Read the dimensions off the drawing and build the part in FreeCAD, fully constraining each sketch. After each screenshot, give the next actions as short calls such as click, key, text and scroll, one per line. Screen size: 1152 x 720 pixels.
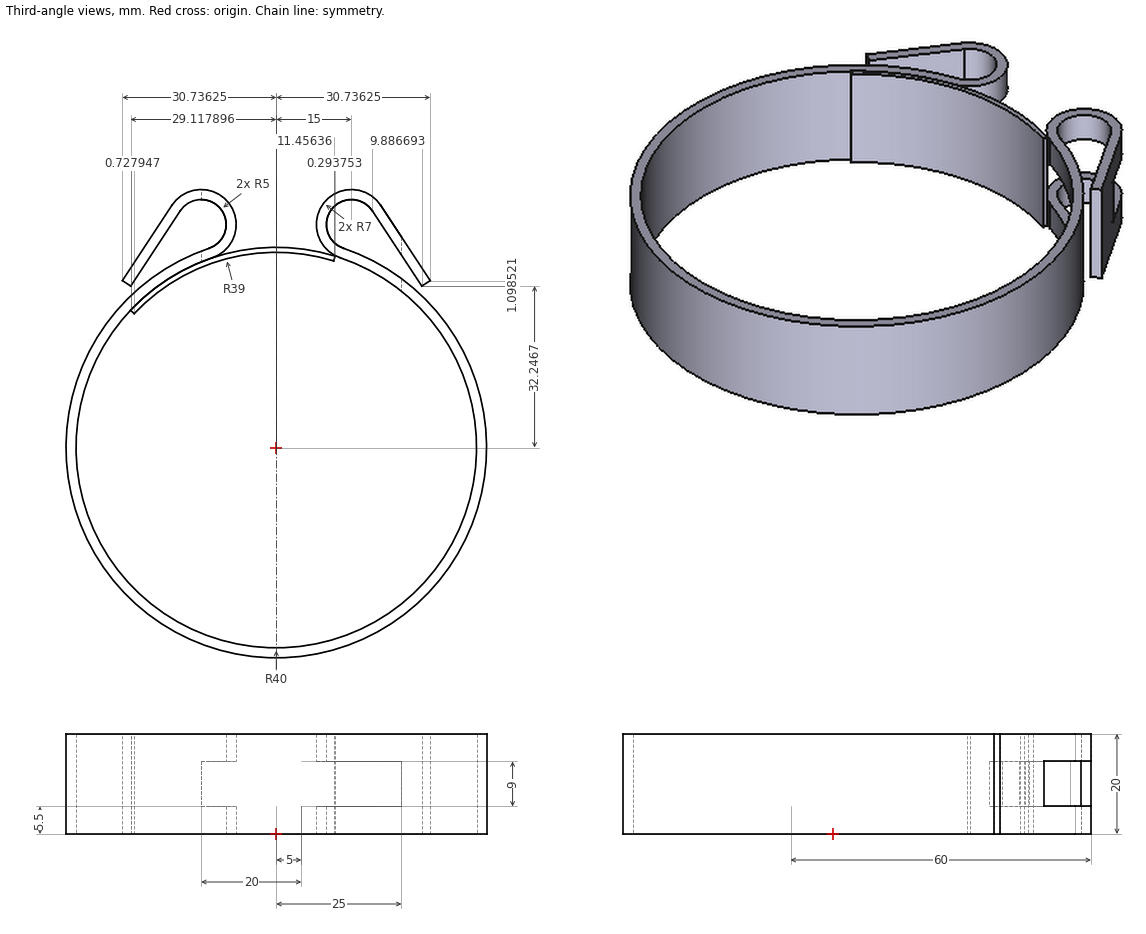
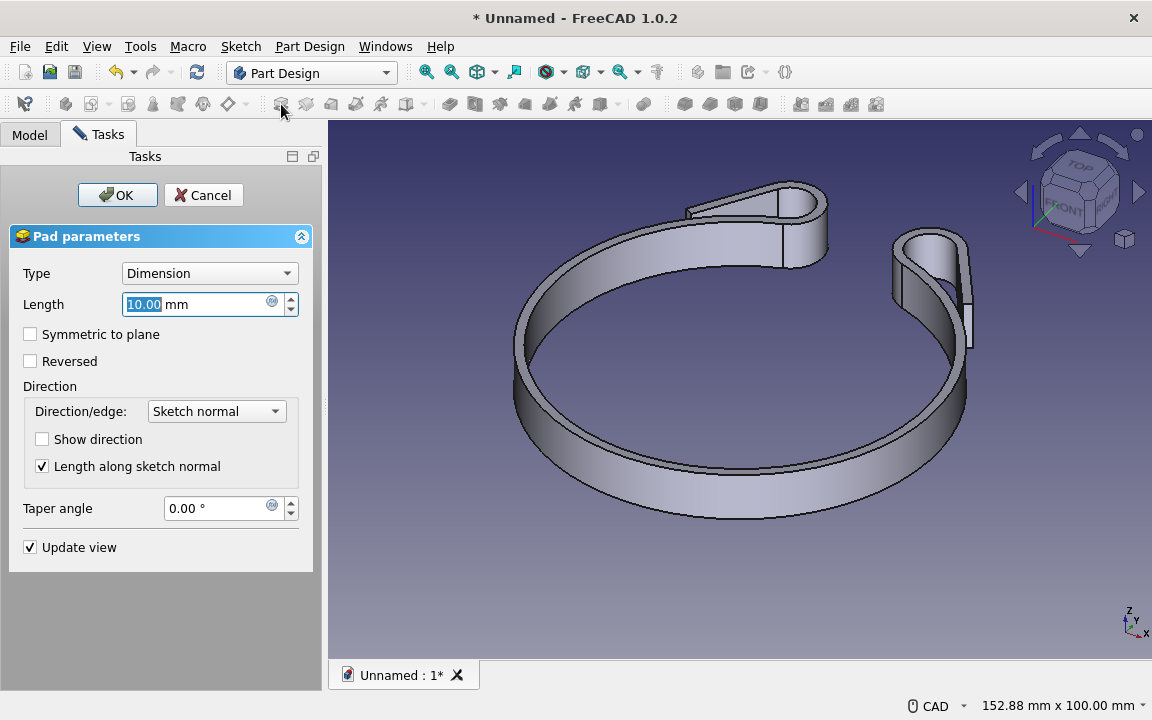
text(20)
key(Tab)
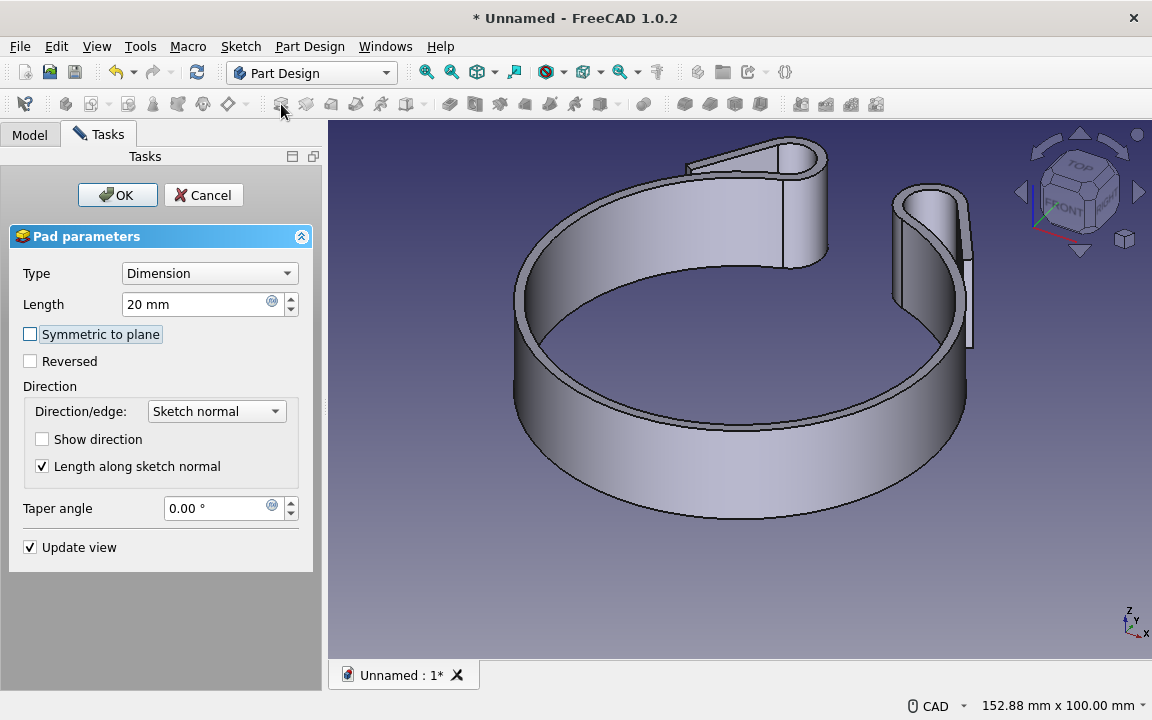
click(118, 195)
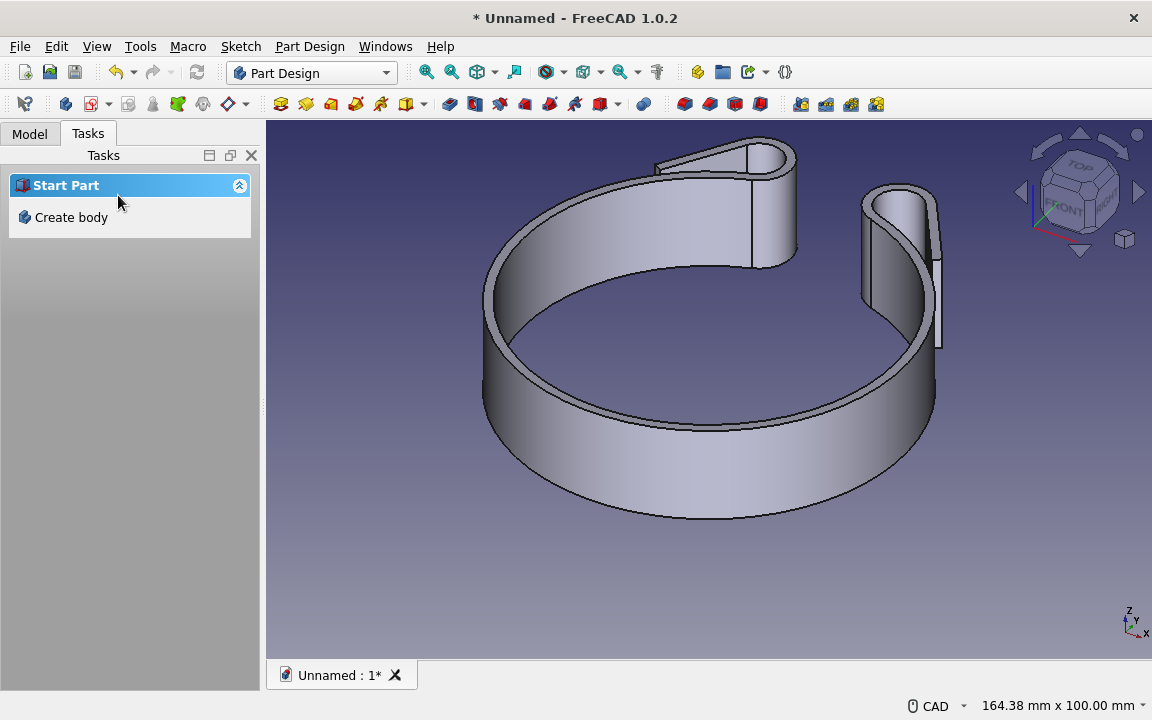
key(v)
key(f)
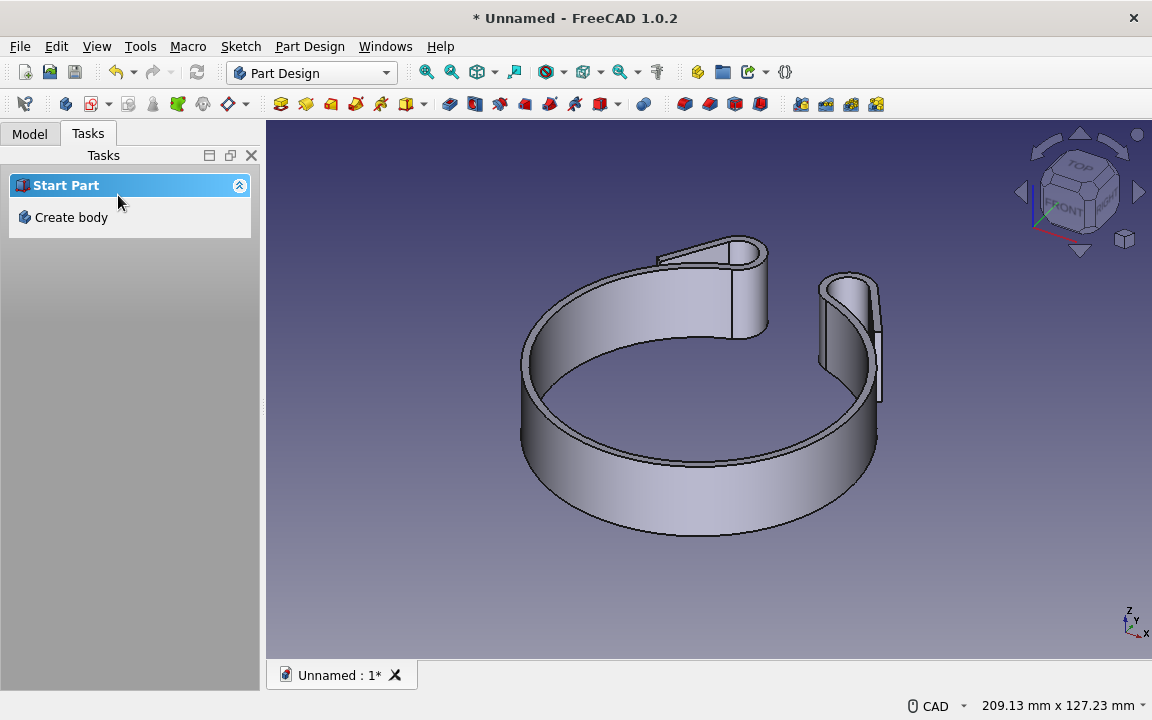
click(90, 104)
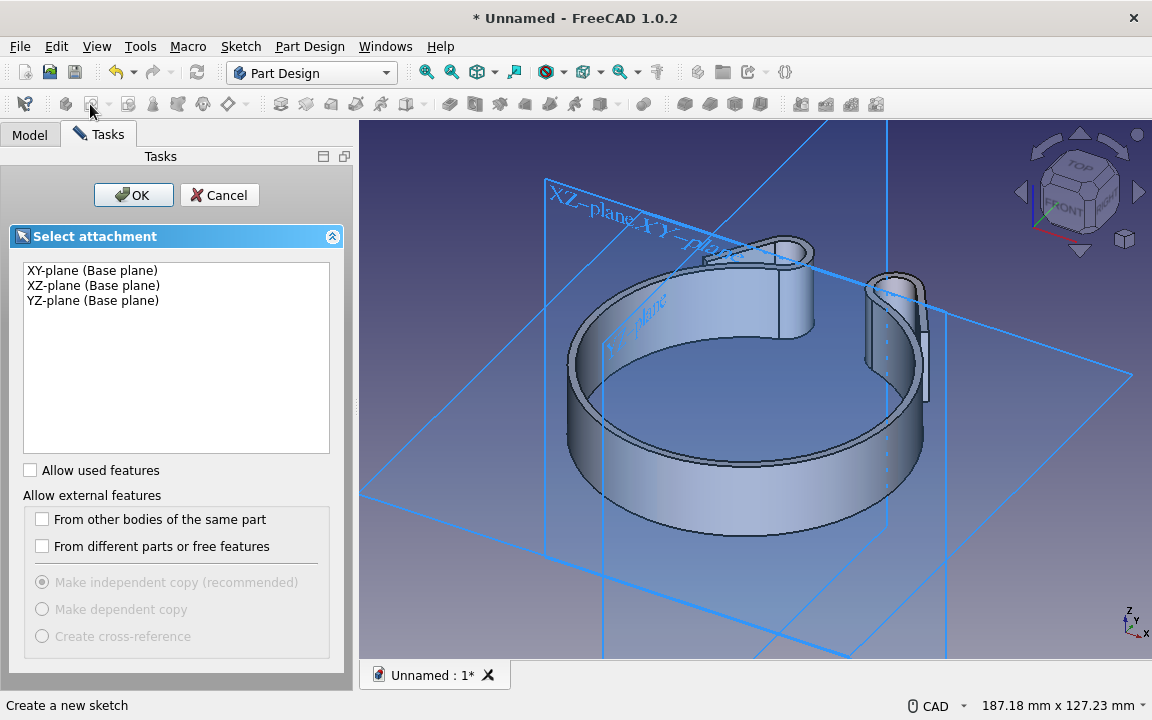
click(84, 286)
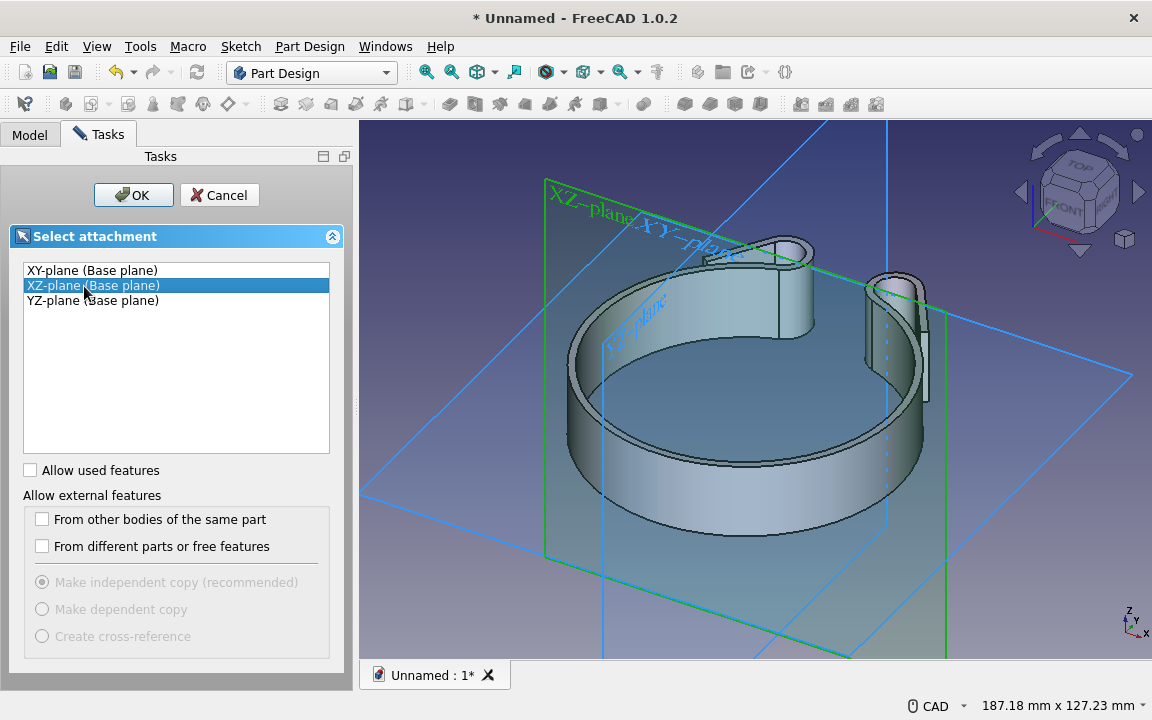
click(134, 195)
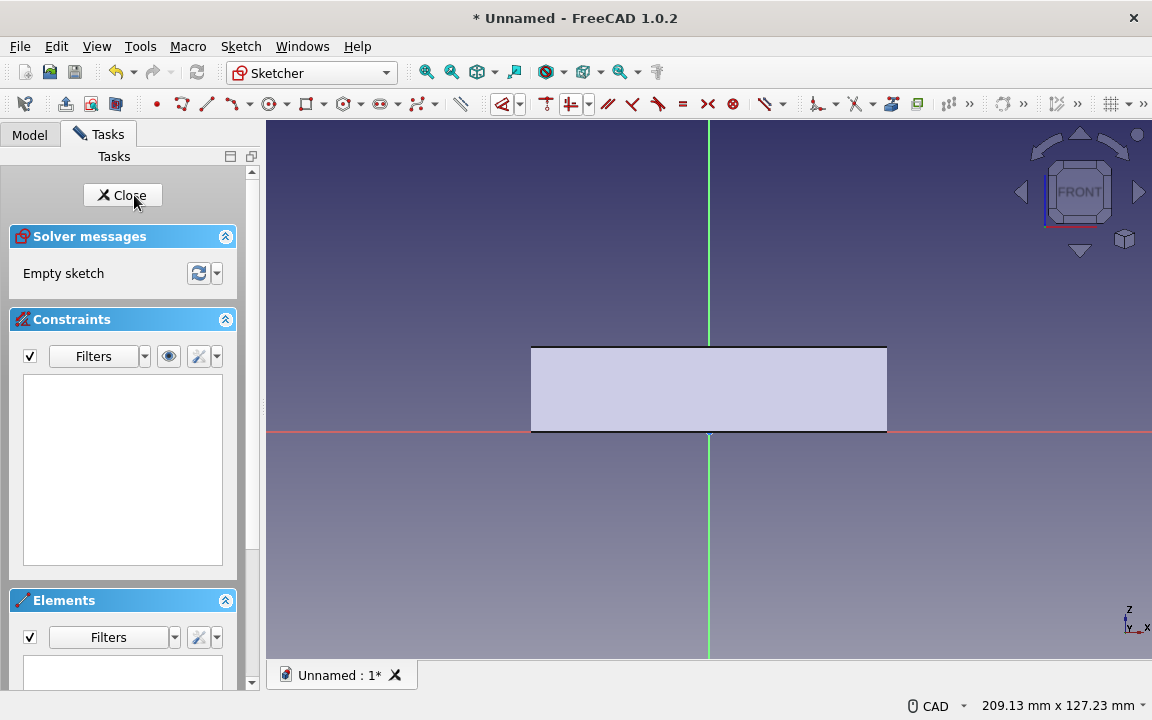
key(q)
key(s)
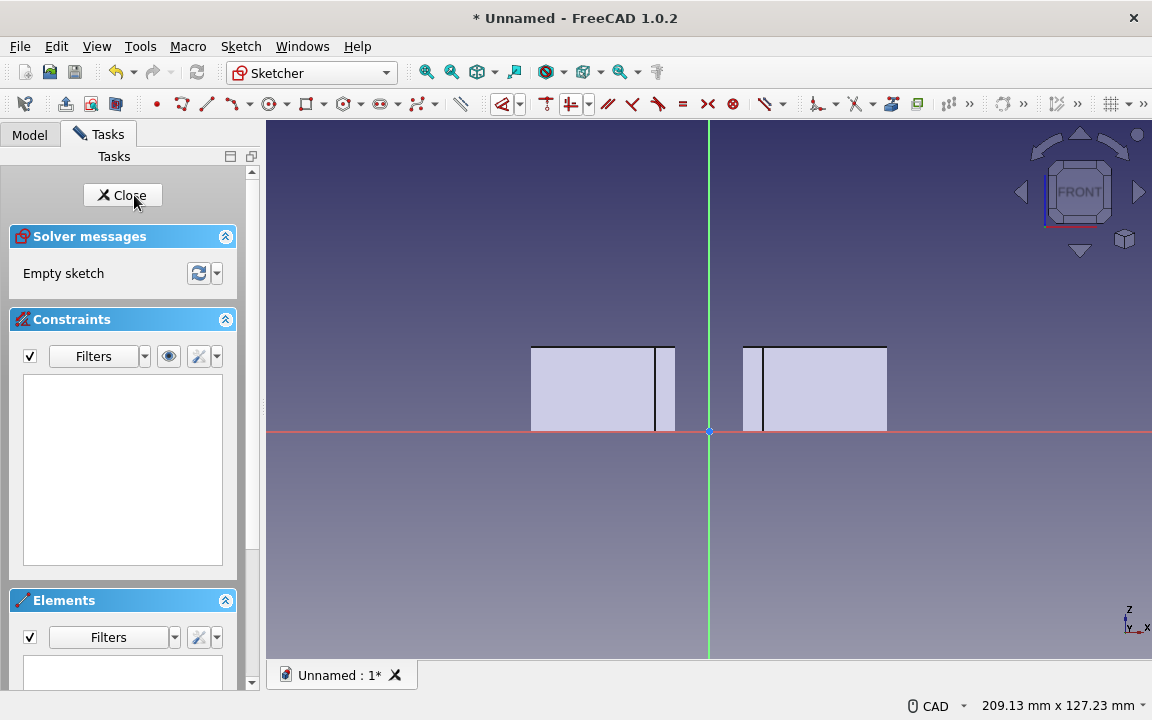
scroll(697, 403, up, 9)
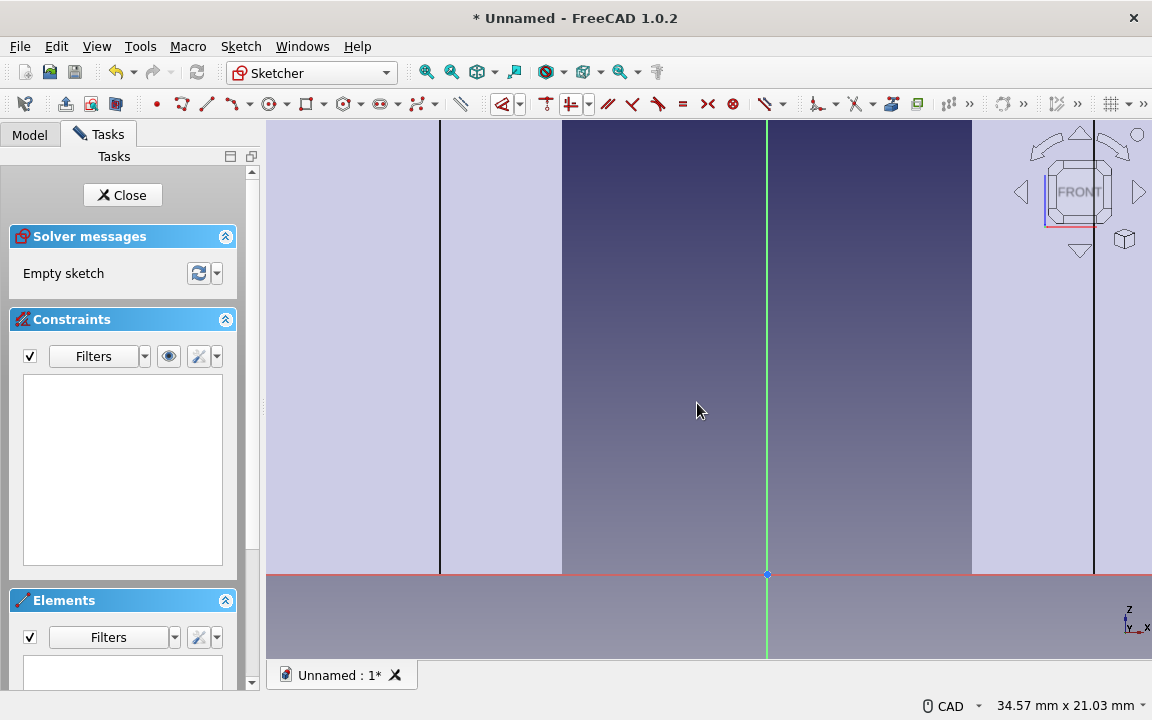
click(306, 104)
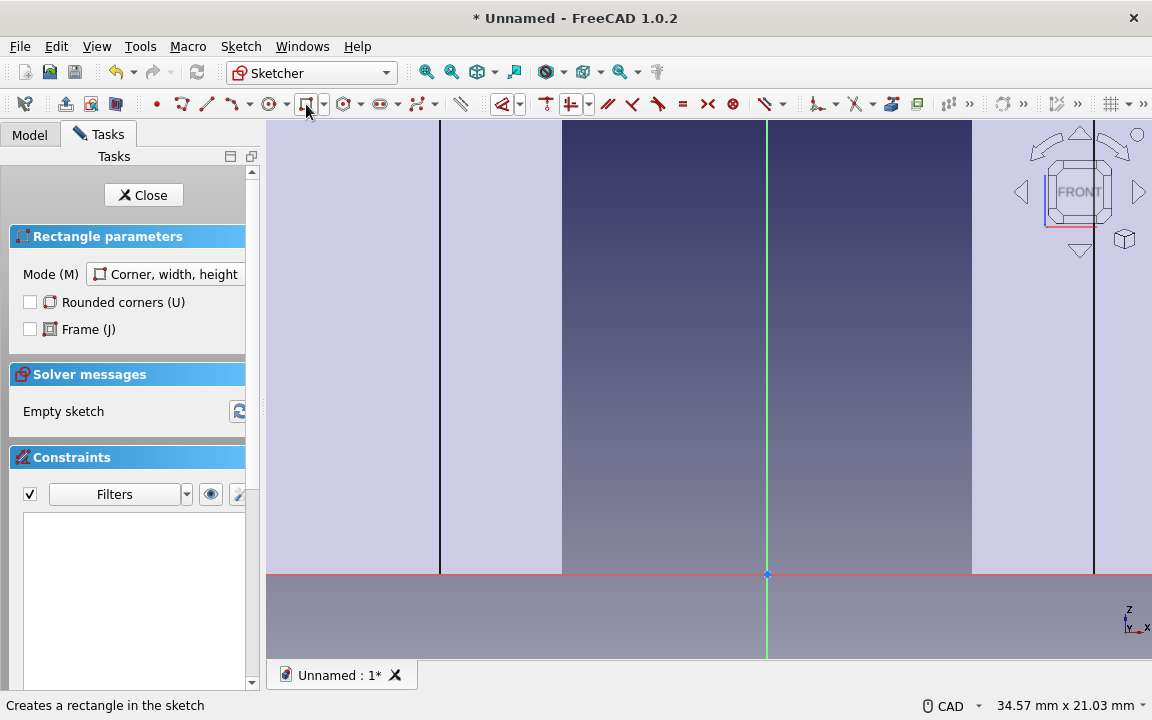
click(383, 203)
move(895, 434)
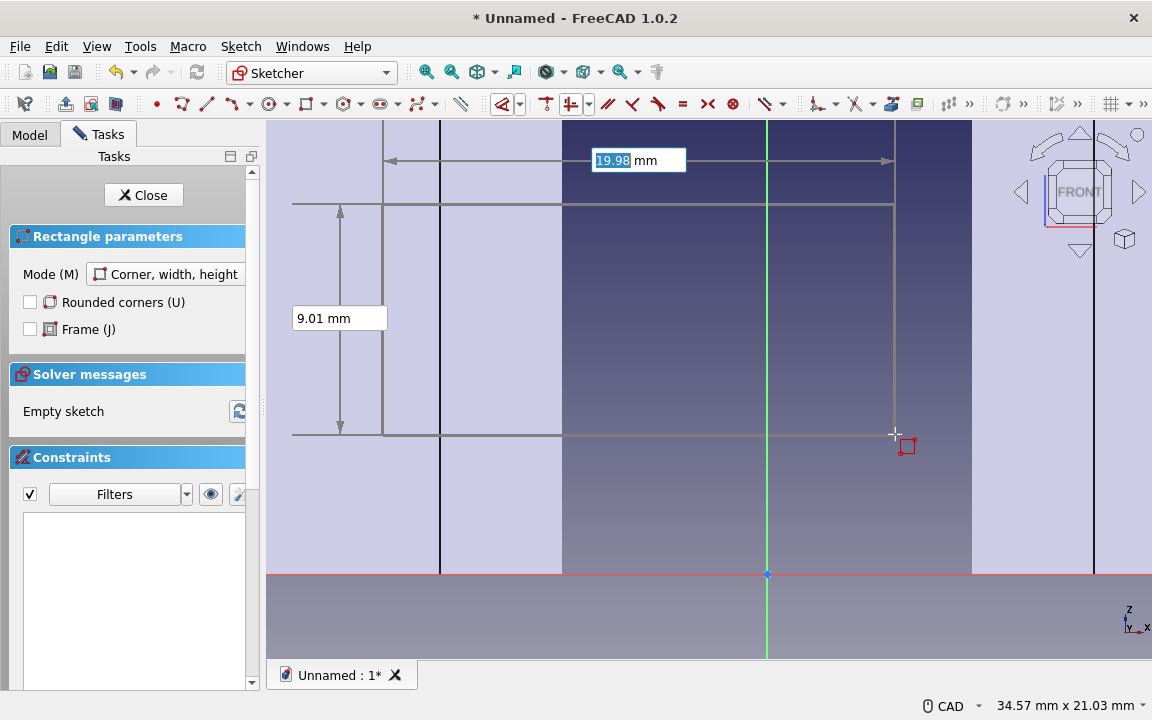
text(20)
key(Tab)
text(9)
key(Return)
key(Escape)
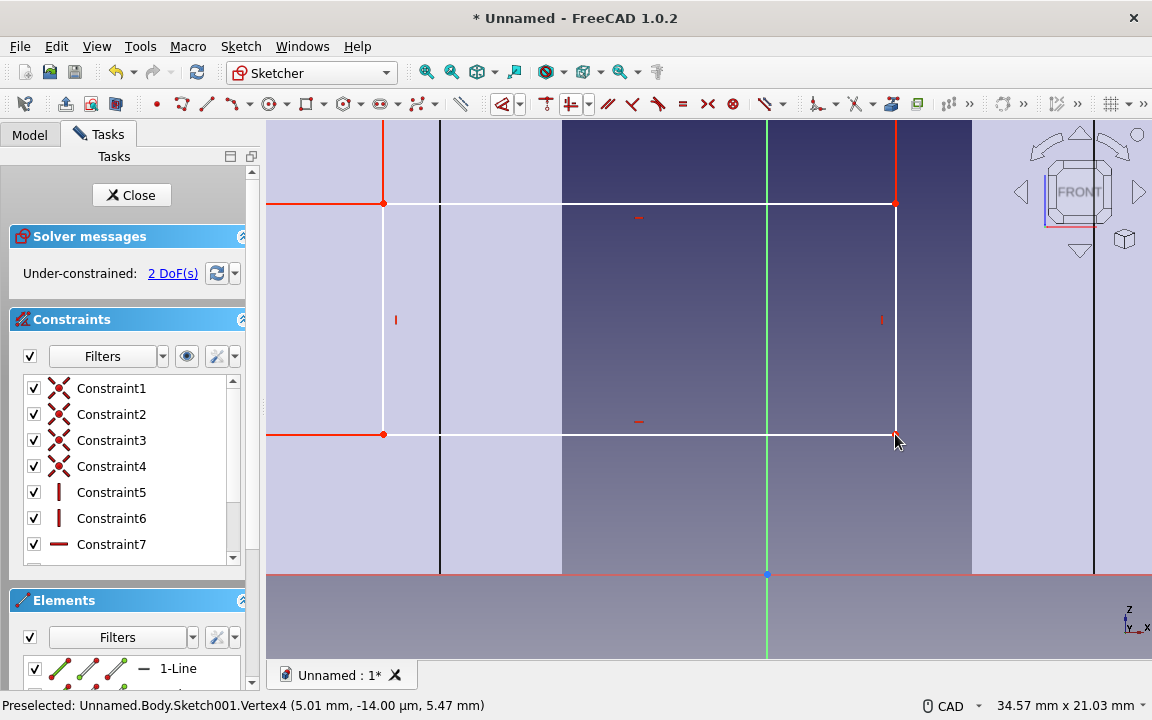
click(896, 435)